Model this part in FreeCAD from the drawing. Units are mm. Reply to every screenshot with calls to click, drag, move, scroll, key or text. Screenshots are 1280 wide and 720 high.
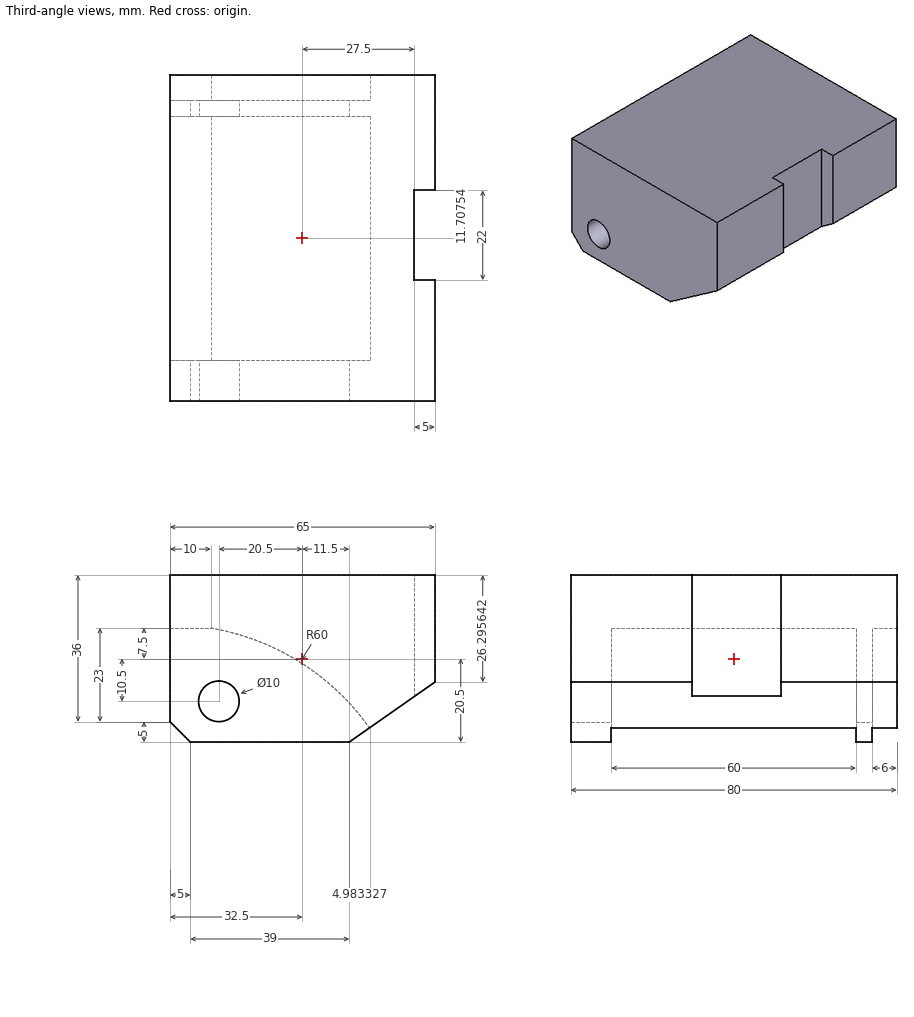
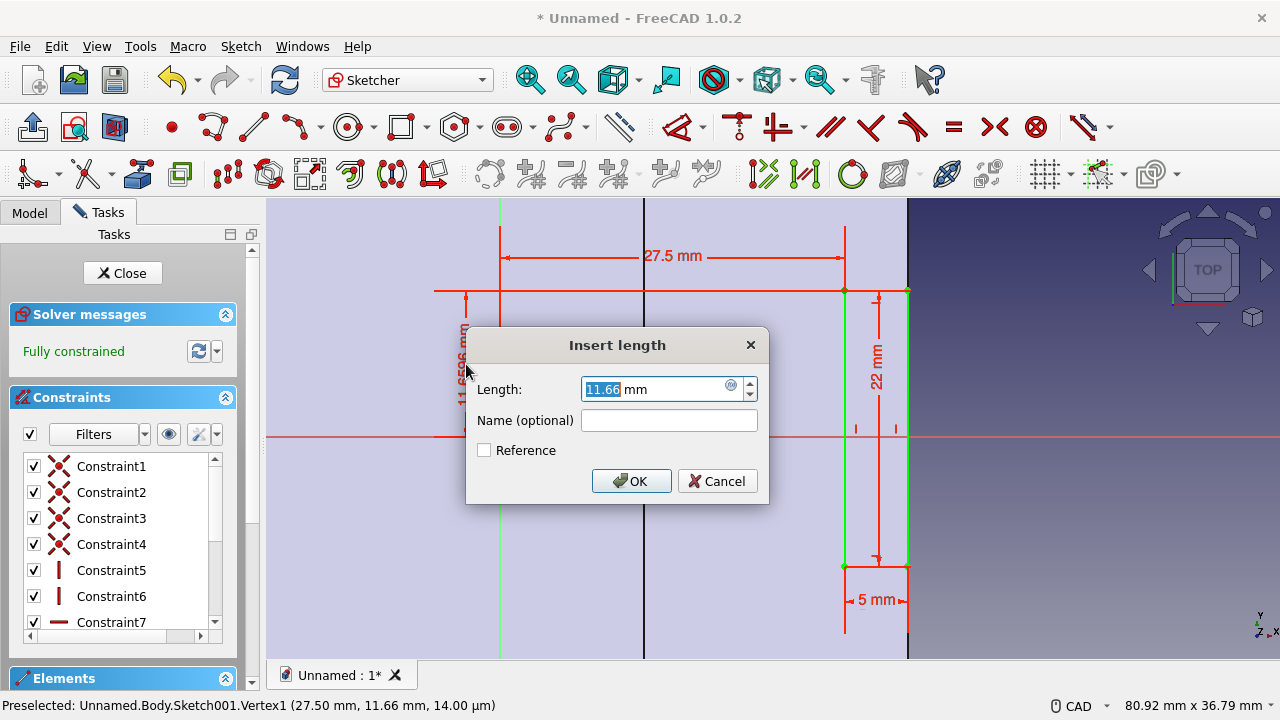
text(11.70754)
key(Return)
key(Escape)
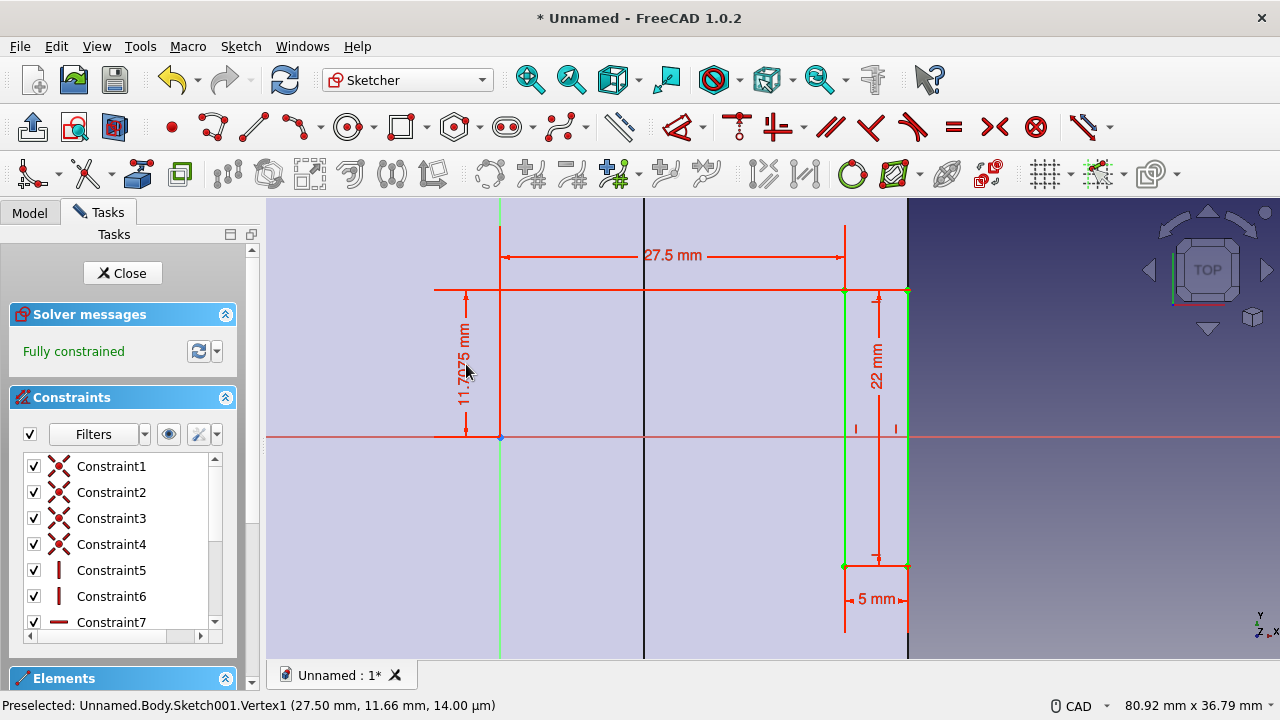
click(123, 273)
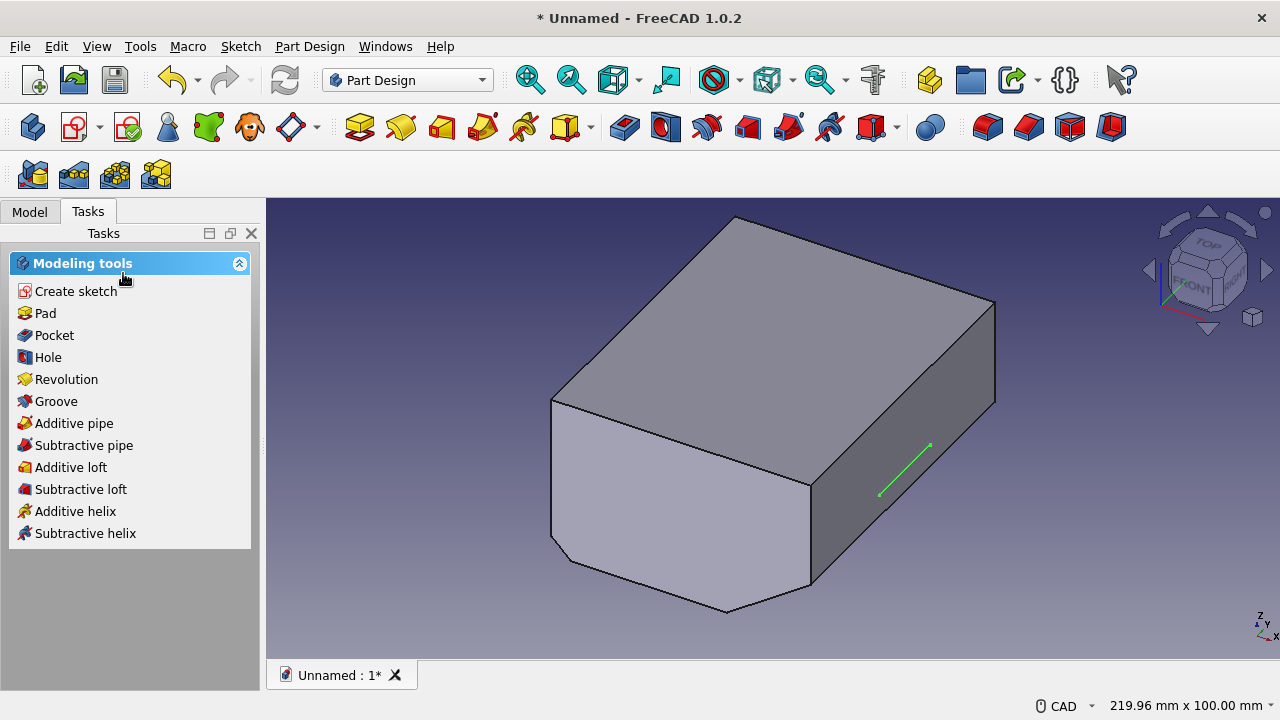
click(625, 128)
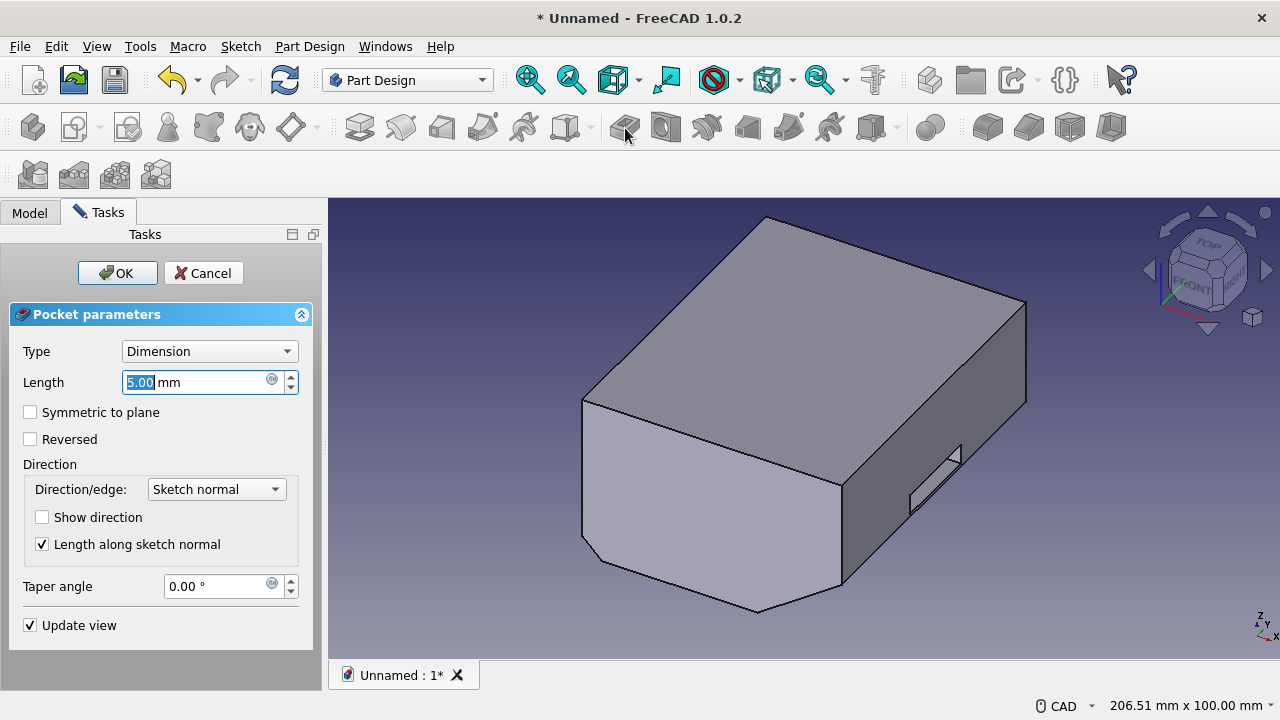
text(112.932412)
key(Tab)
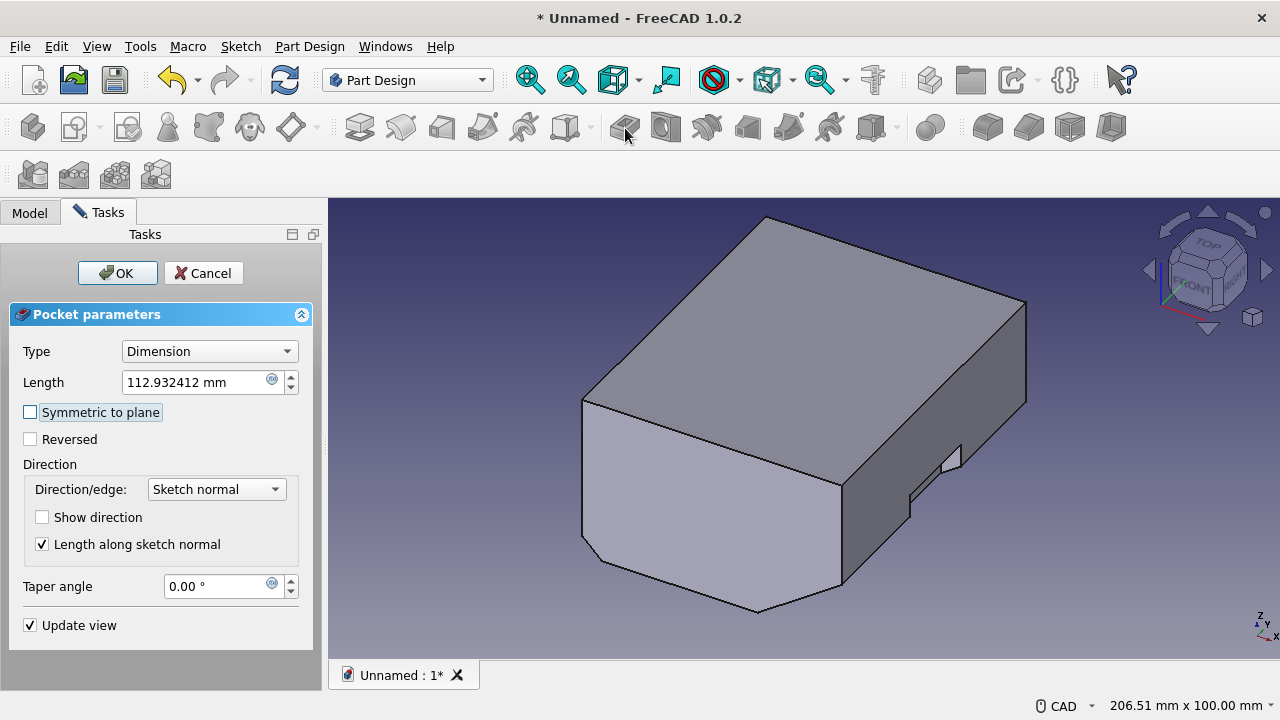
click(31, 412)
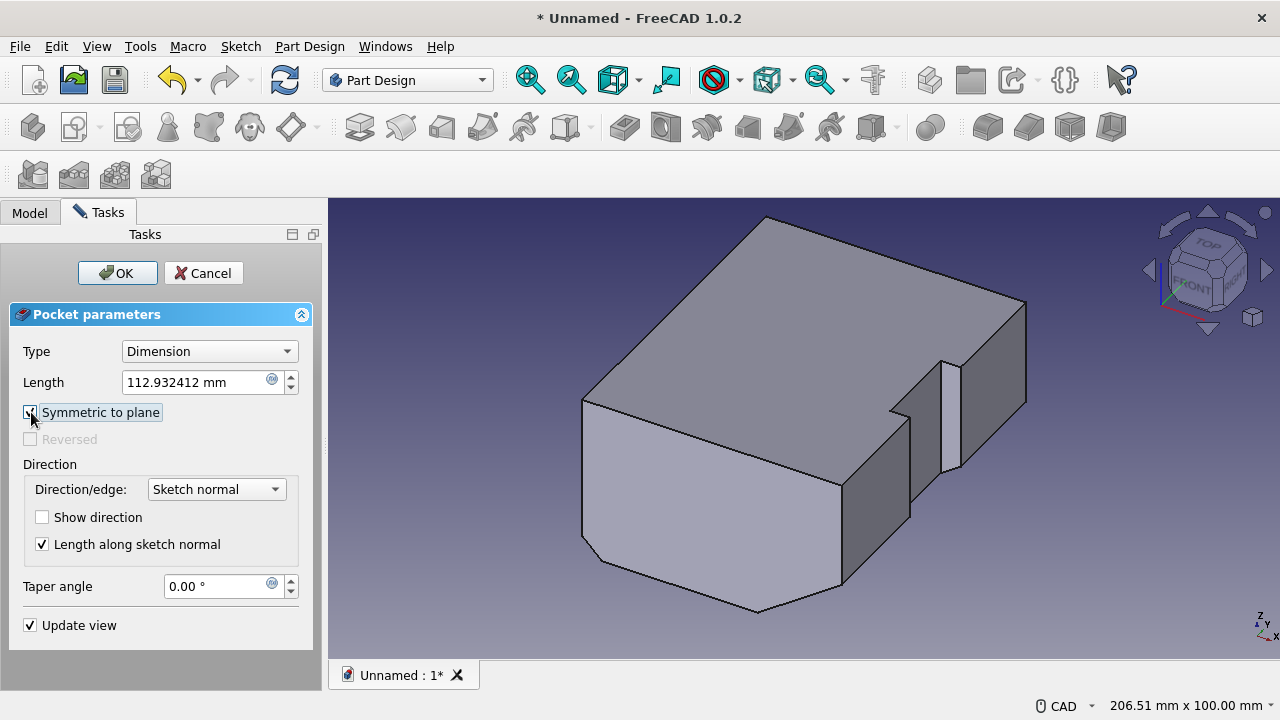
click(118, 273)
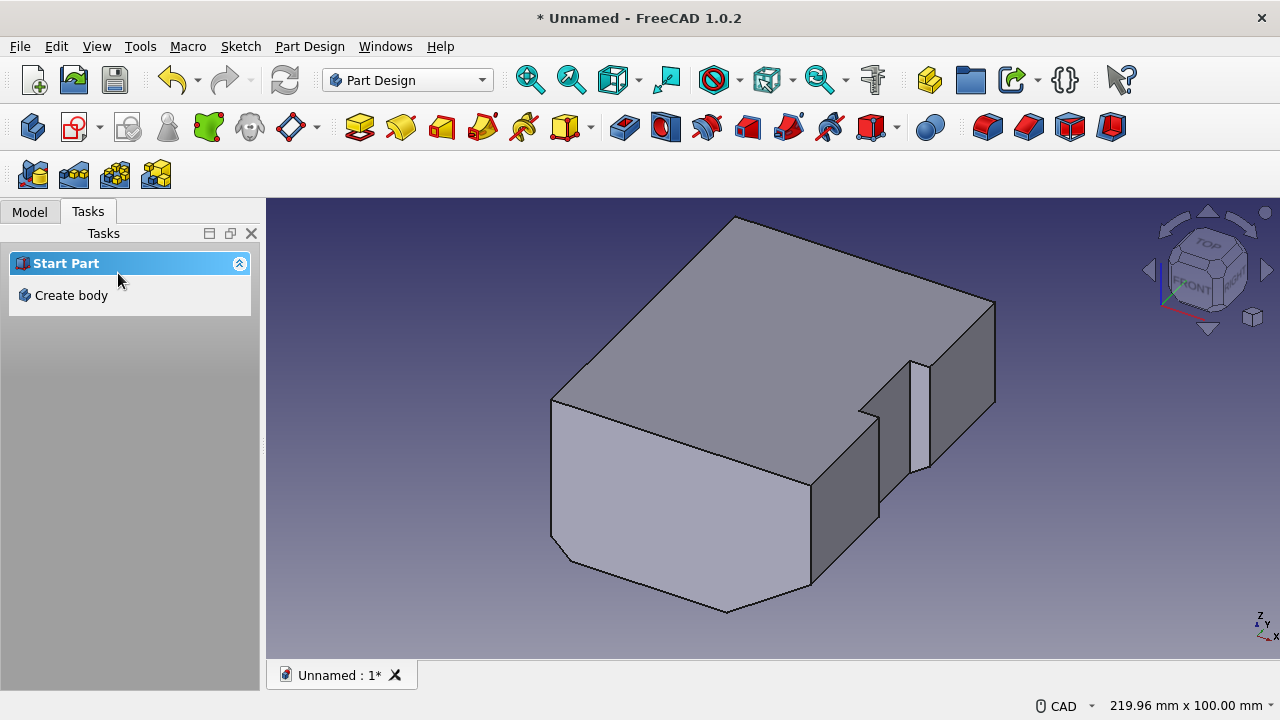
key(4)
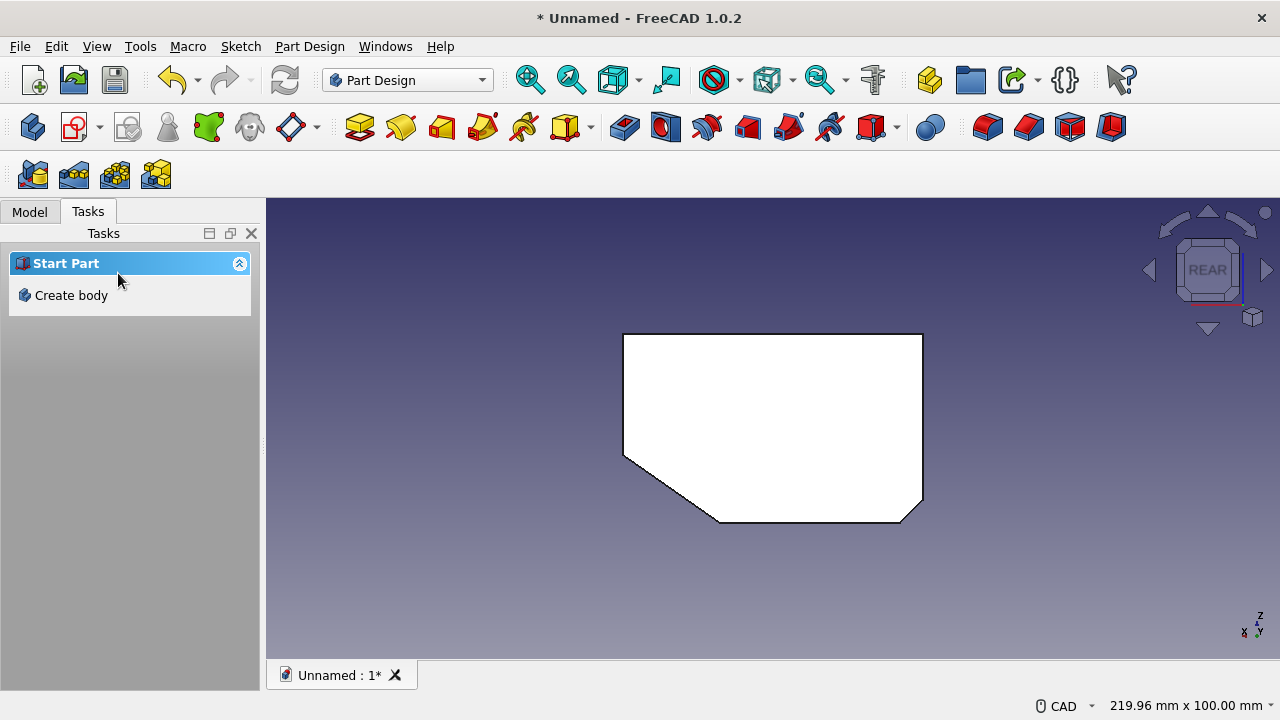
key(v)
key(f)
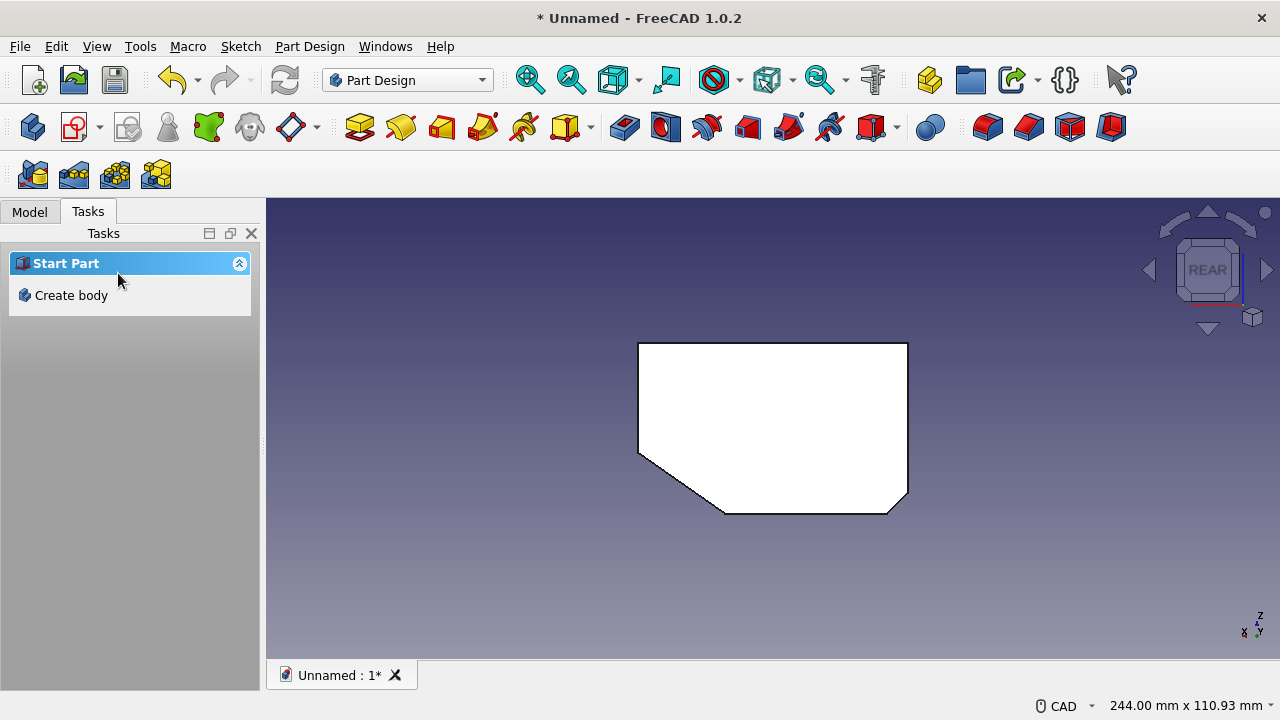
click(773, 428)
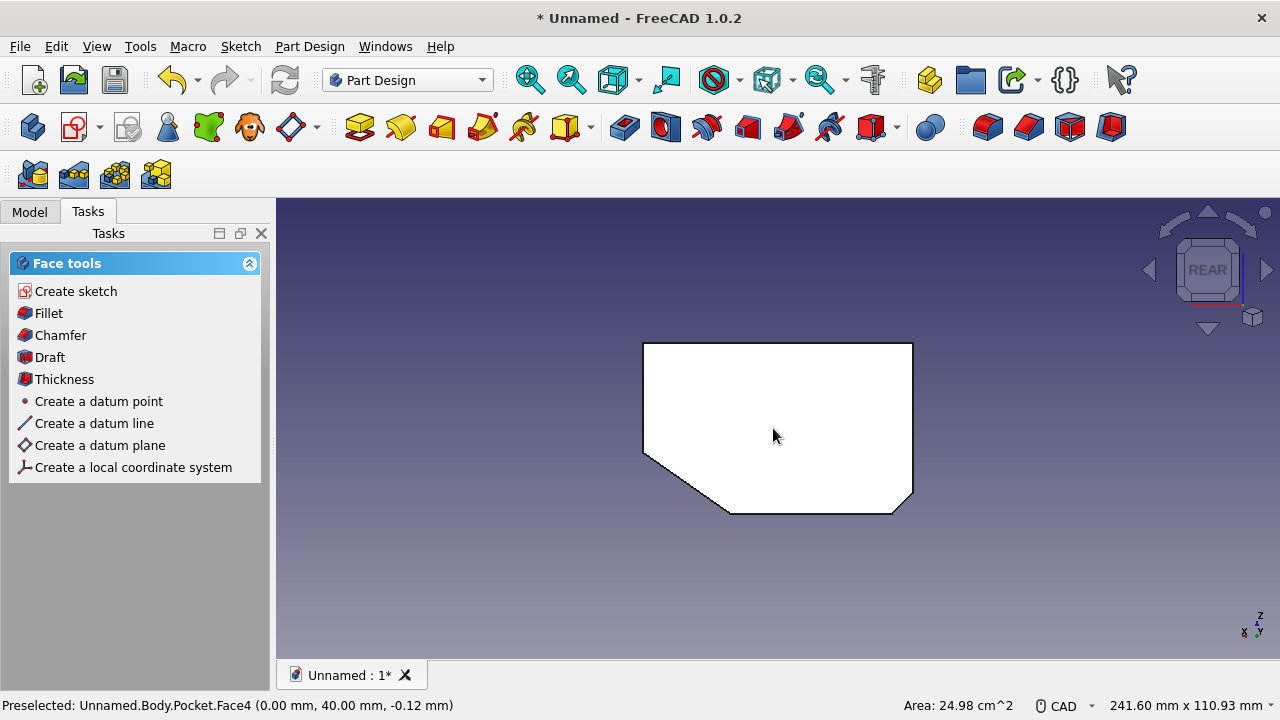
click(74, 128)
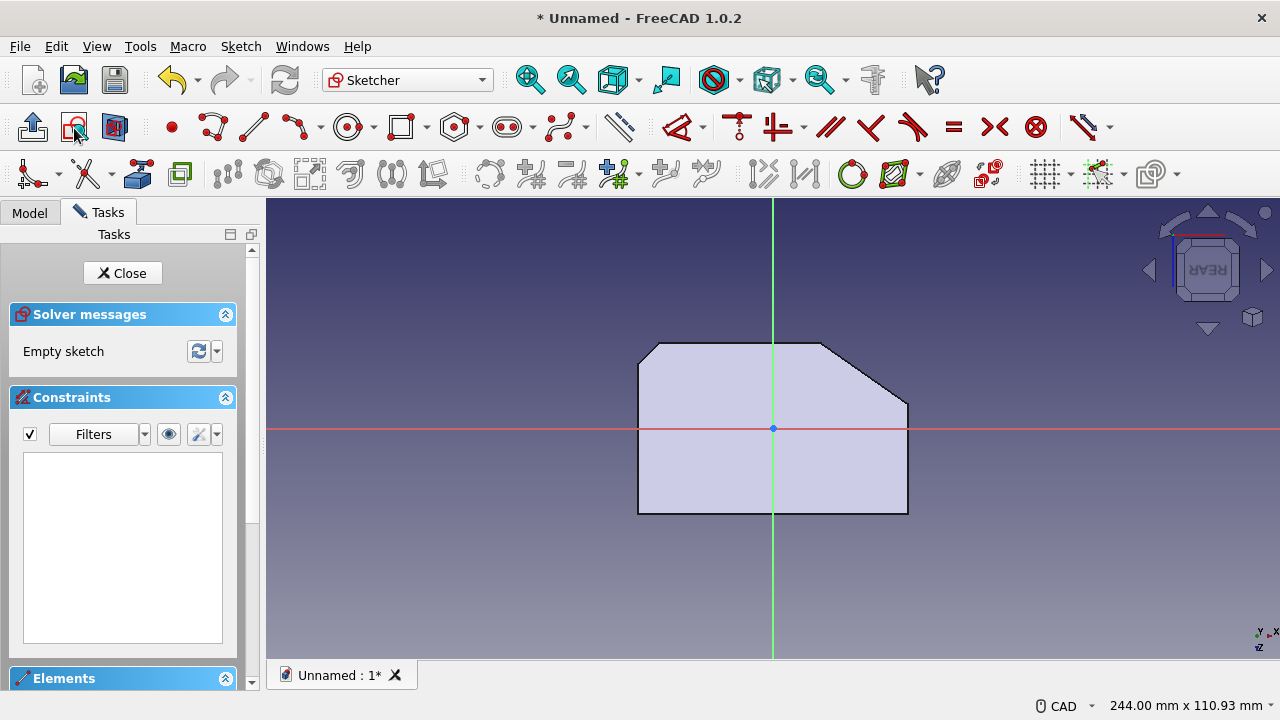
scroll(768, 379, up, 4)